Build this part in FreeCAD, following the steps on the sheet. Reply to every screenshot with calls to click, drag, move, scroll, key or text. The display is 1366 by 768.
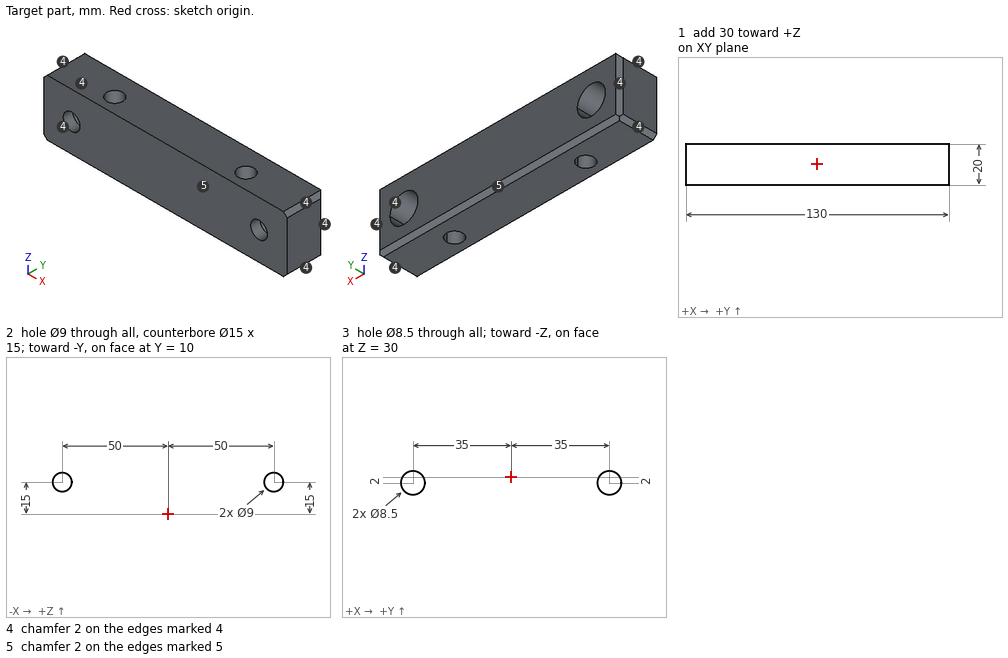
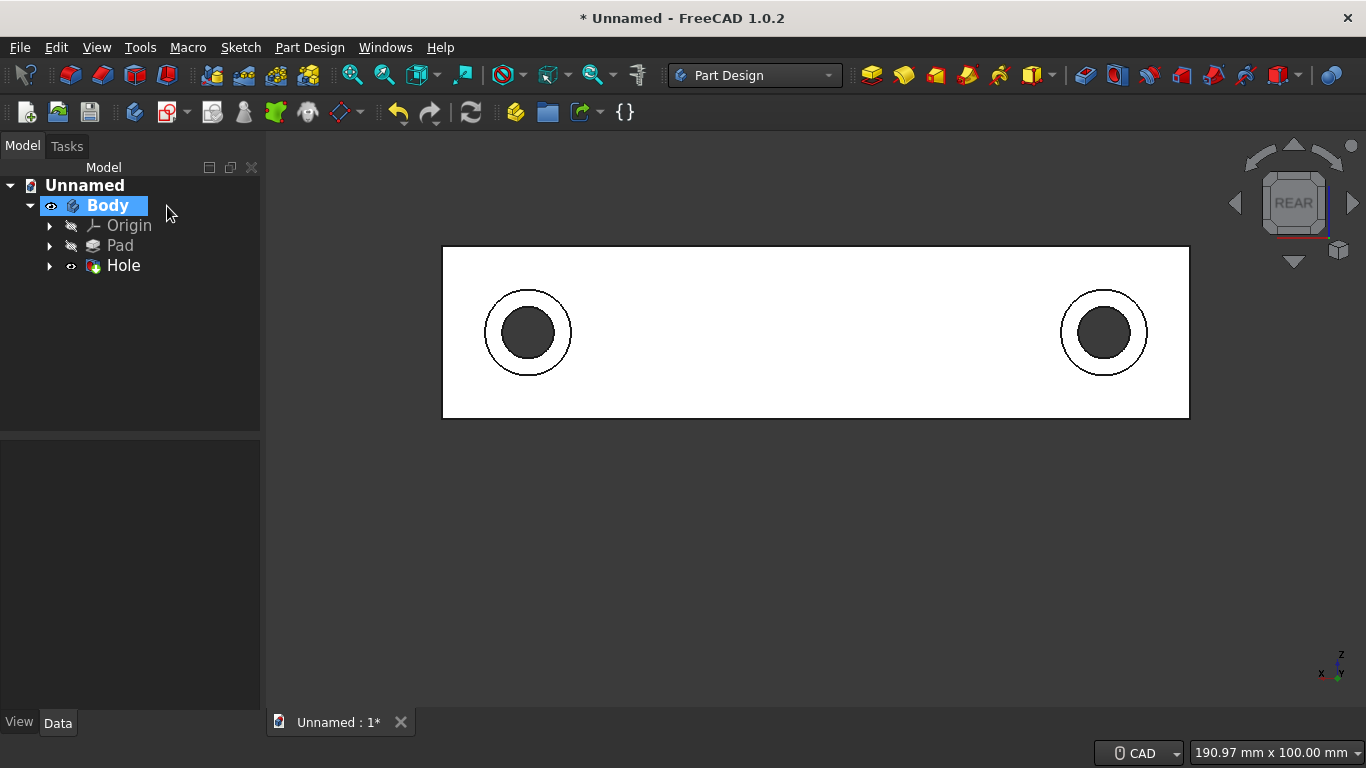
key(0)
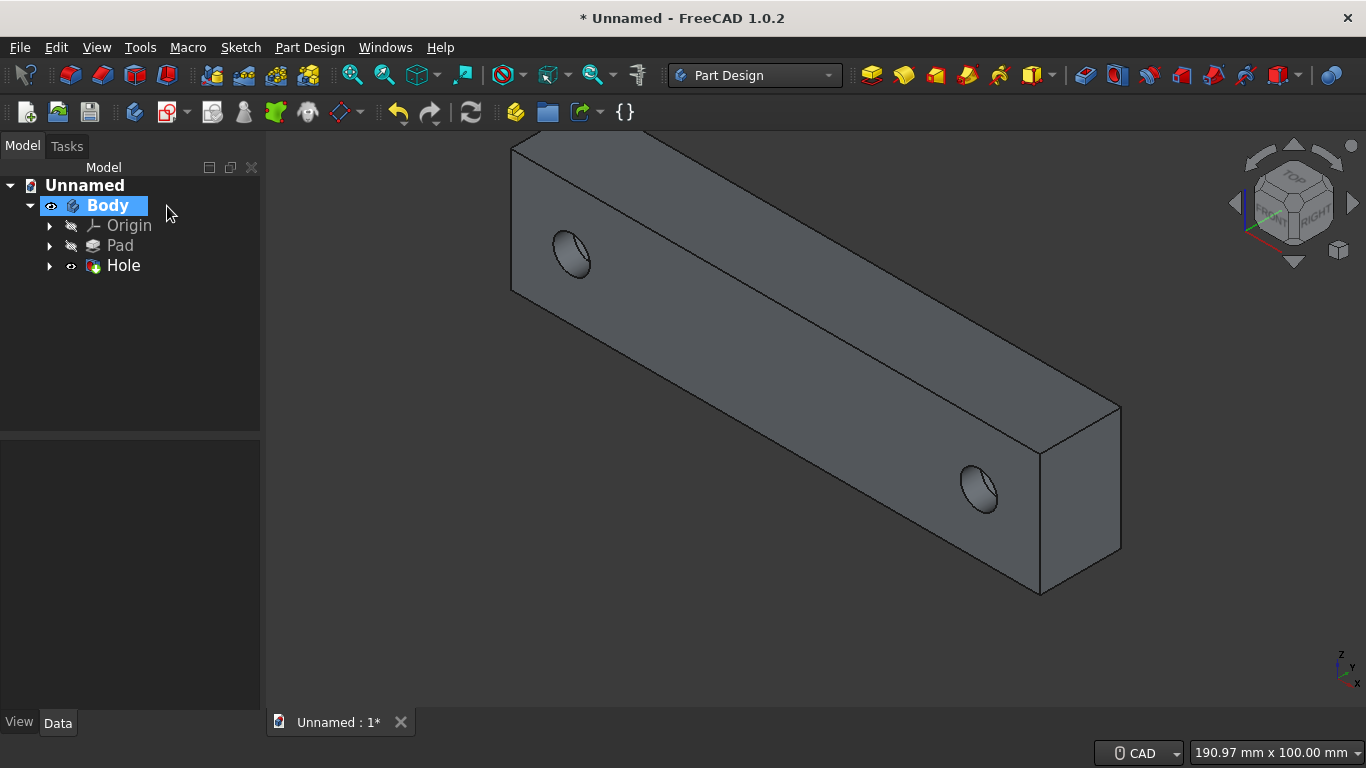
key(v)
key(f)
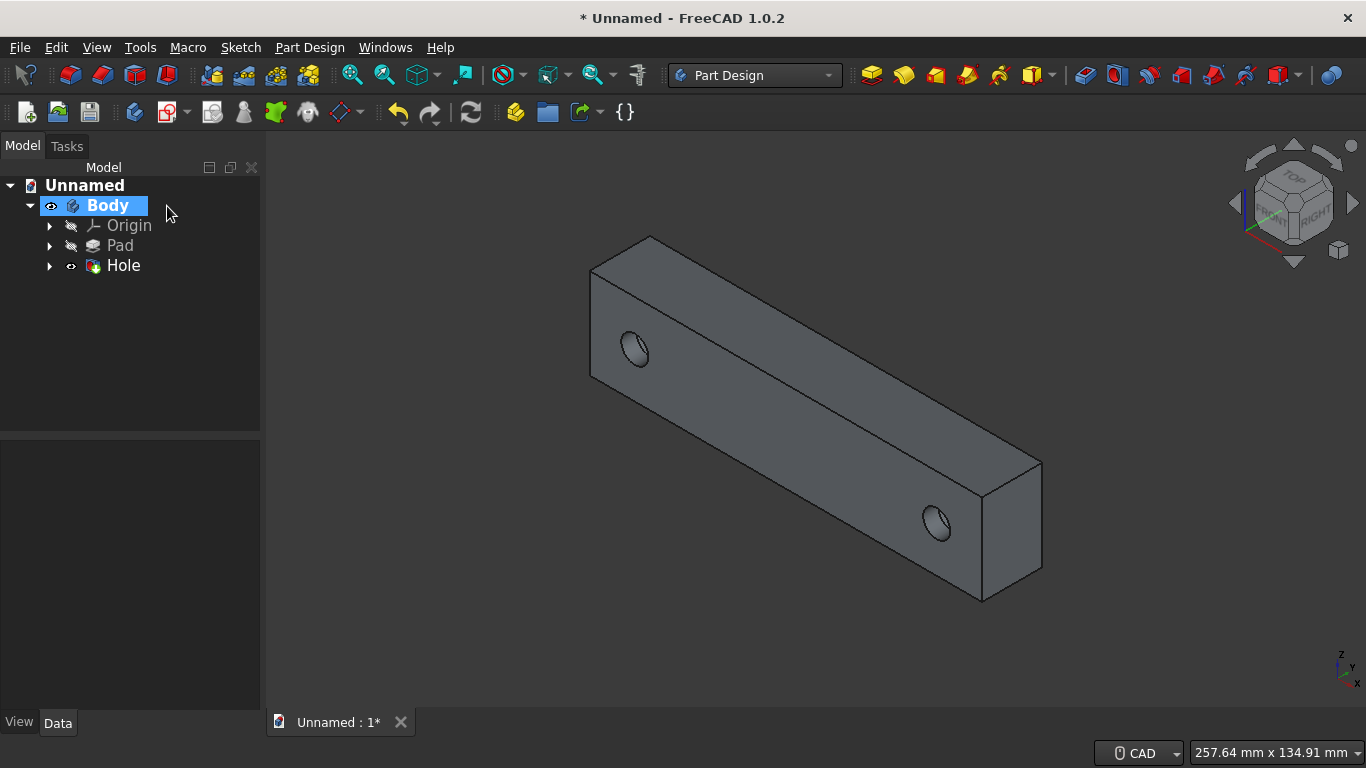
click(928, 430)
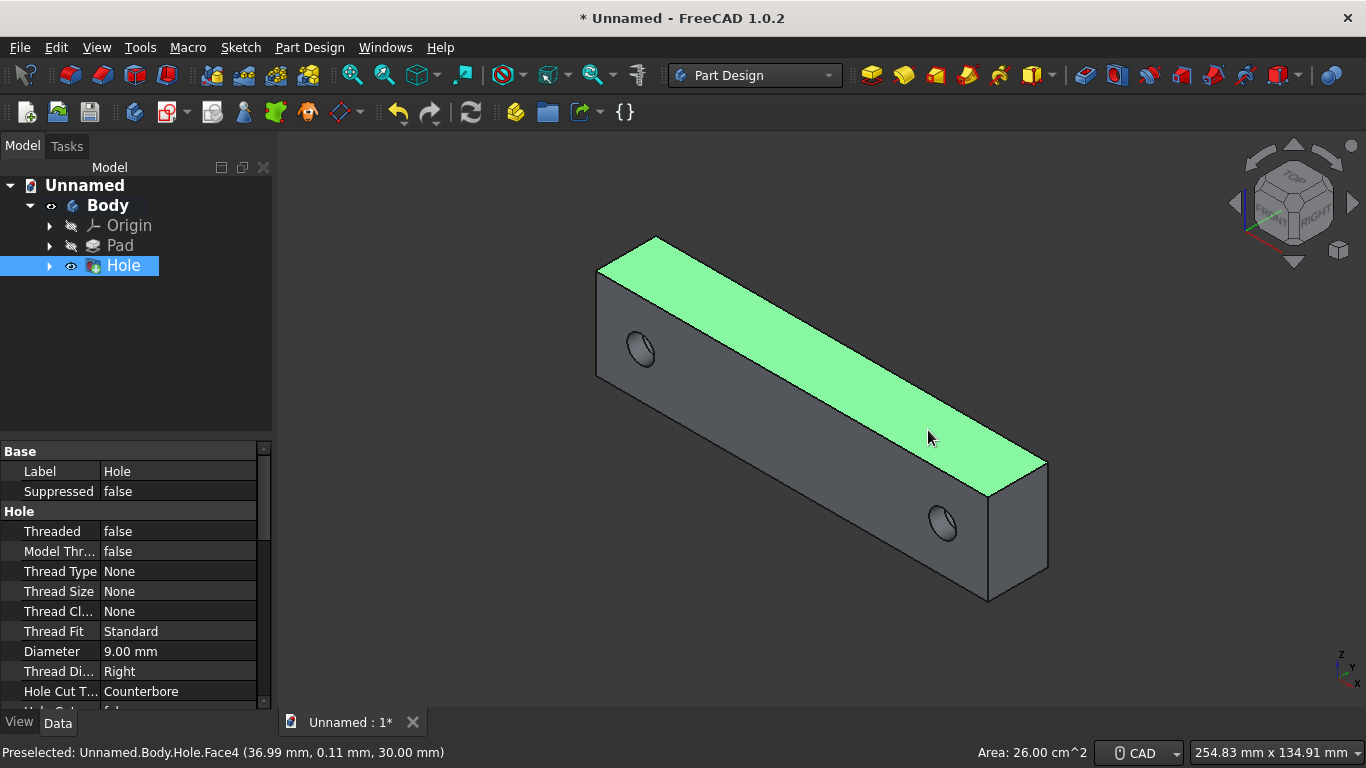
click(168, 112)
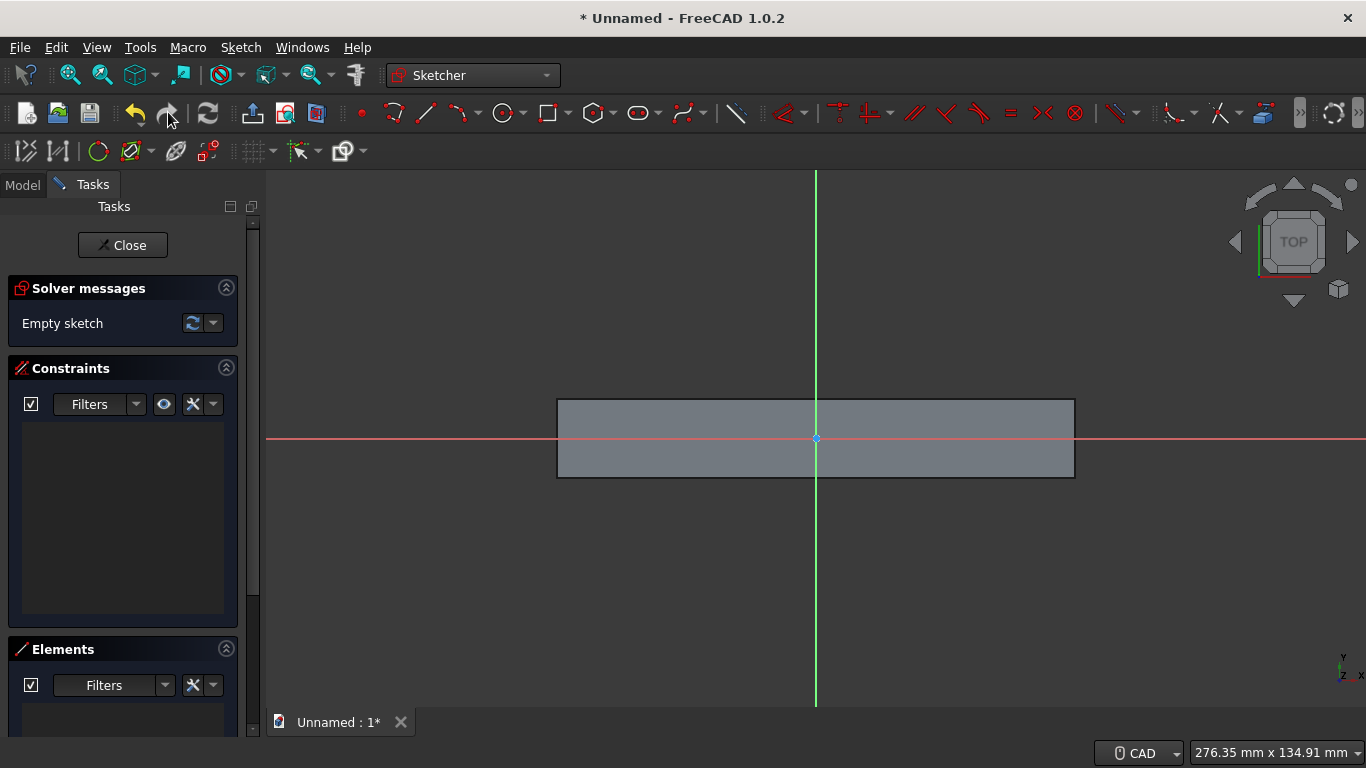
scroll(872, 453, up, 4)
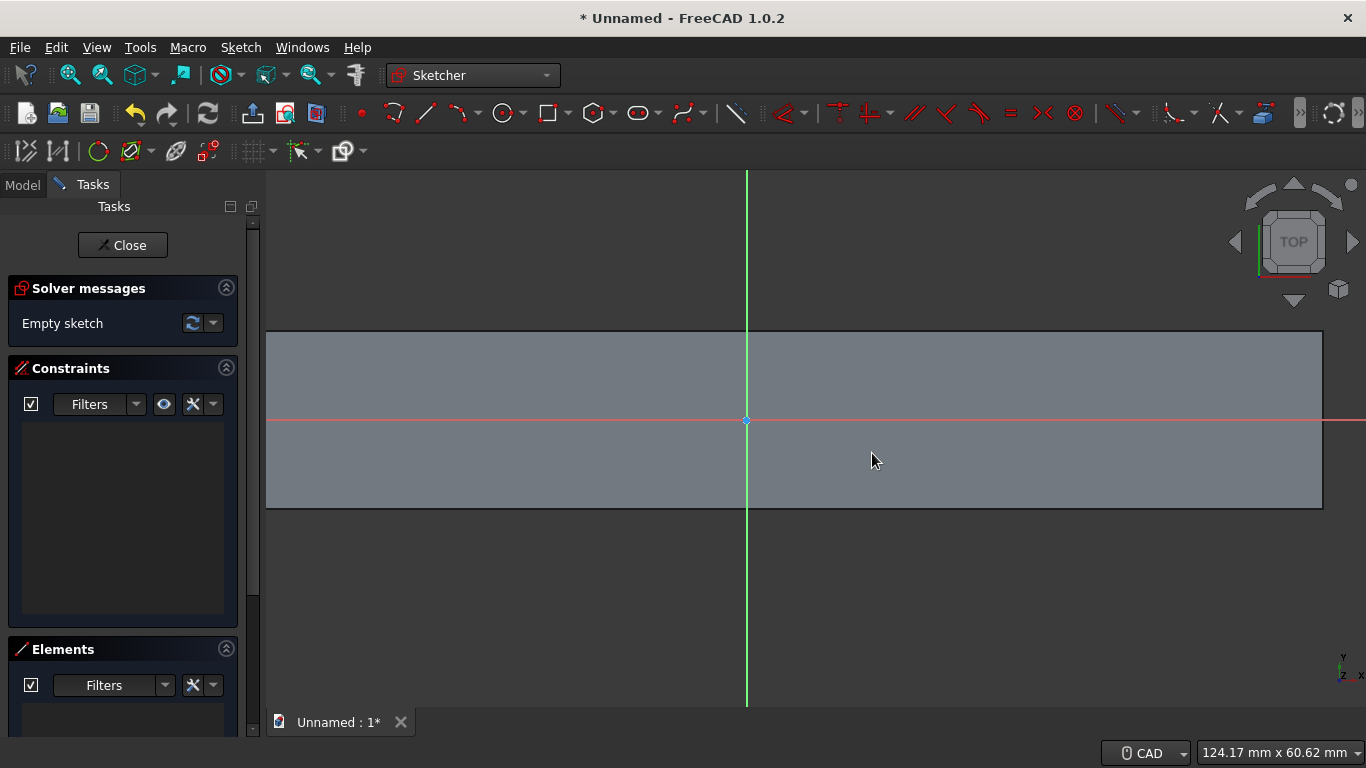
click(504, 114)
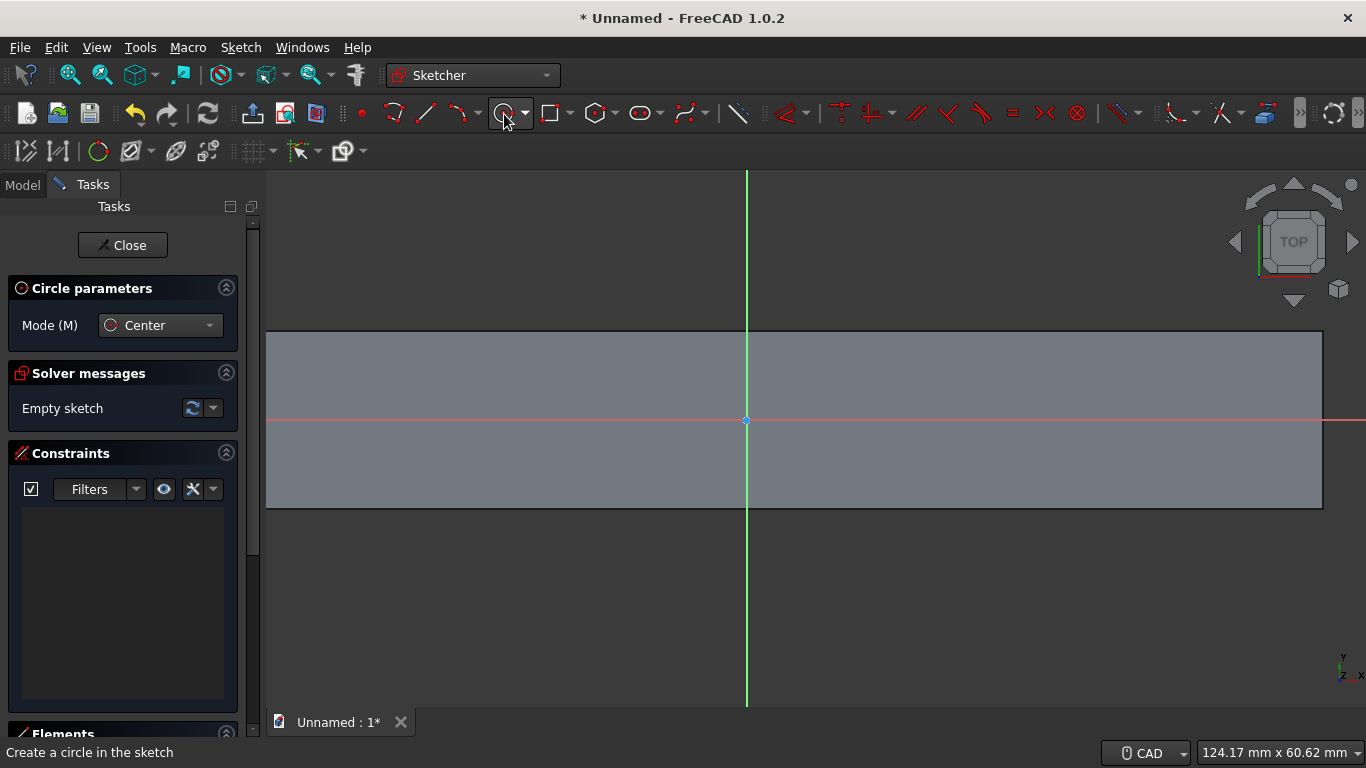
click(437, 438)
move(463, 464)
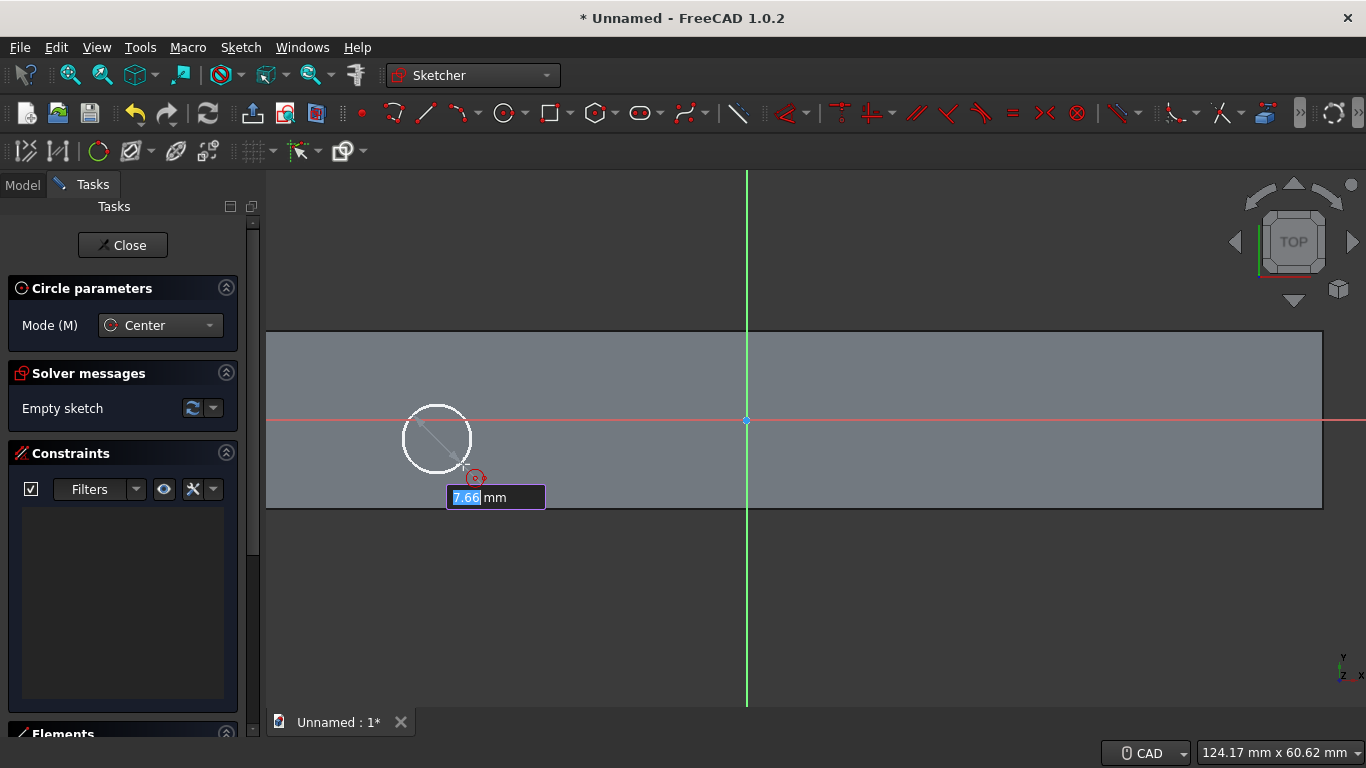
text(8.5)
key(Return)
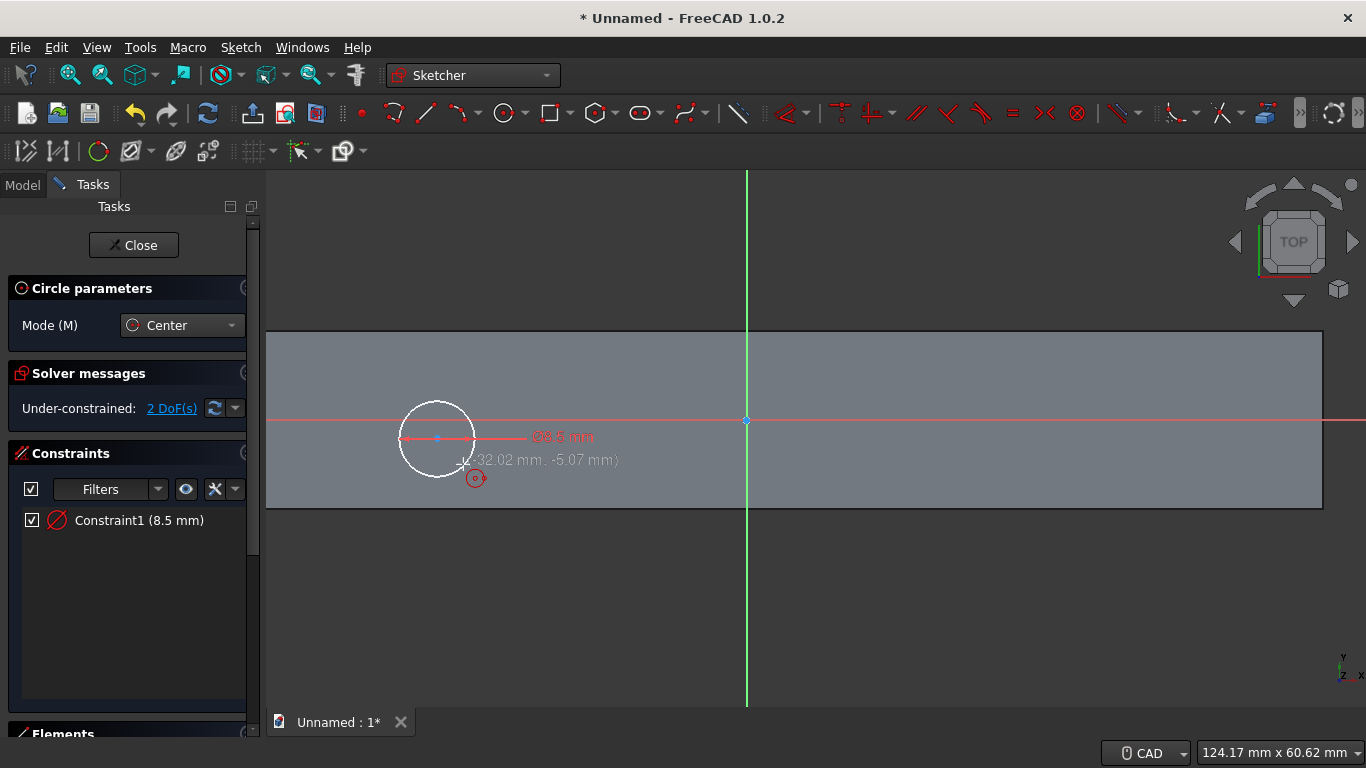
click(1057, 438)
move(1083, 464)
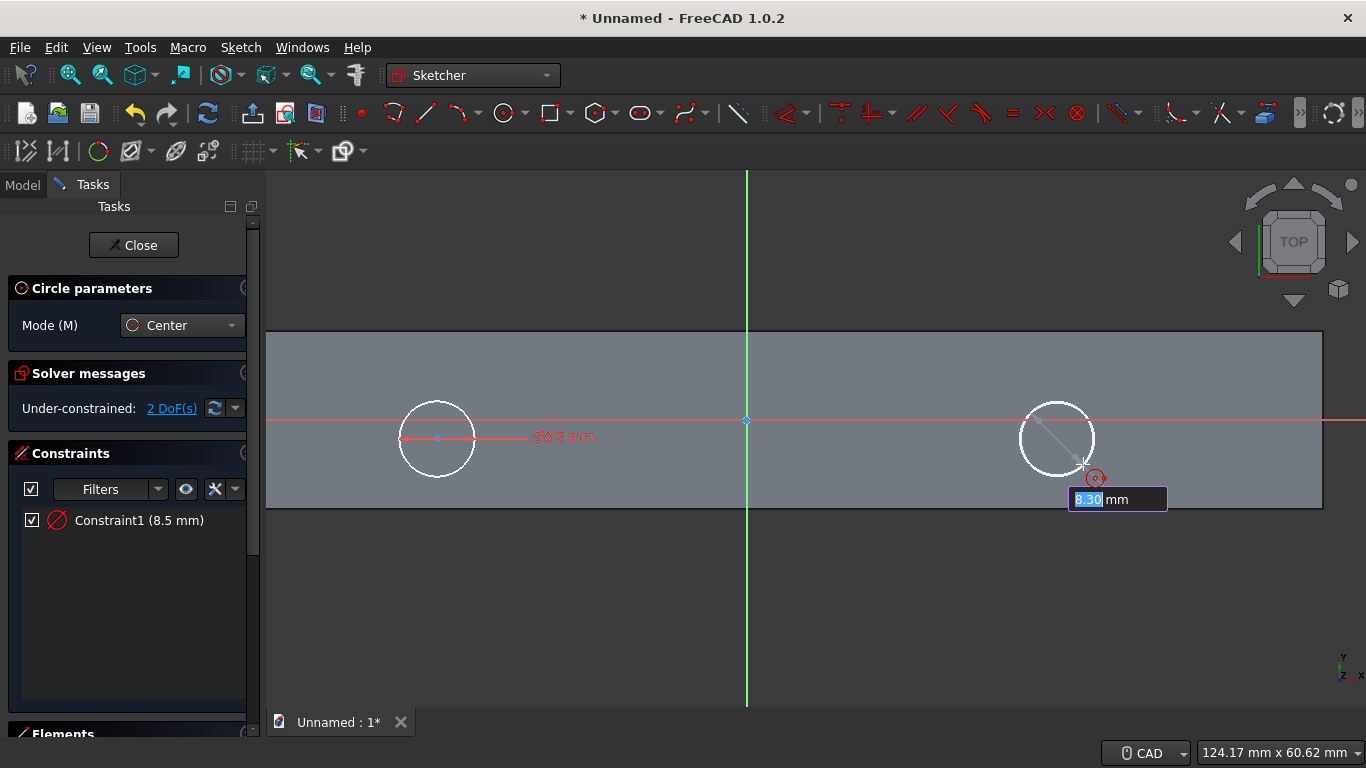
text(8.5)
key(Return)
key(Escape)